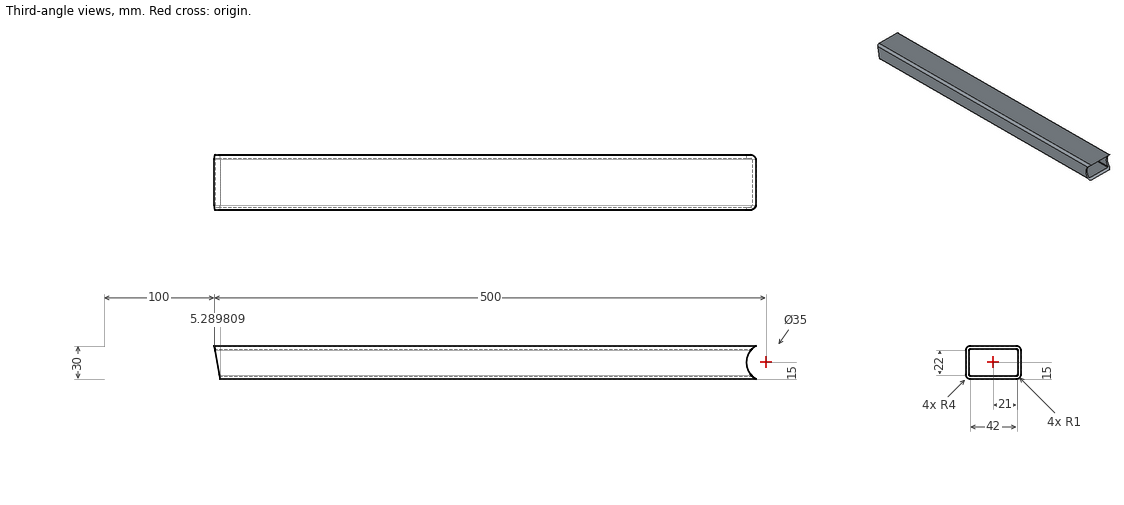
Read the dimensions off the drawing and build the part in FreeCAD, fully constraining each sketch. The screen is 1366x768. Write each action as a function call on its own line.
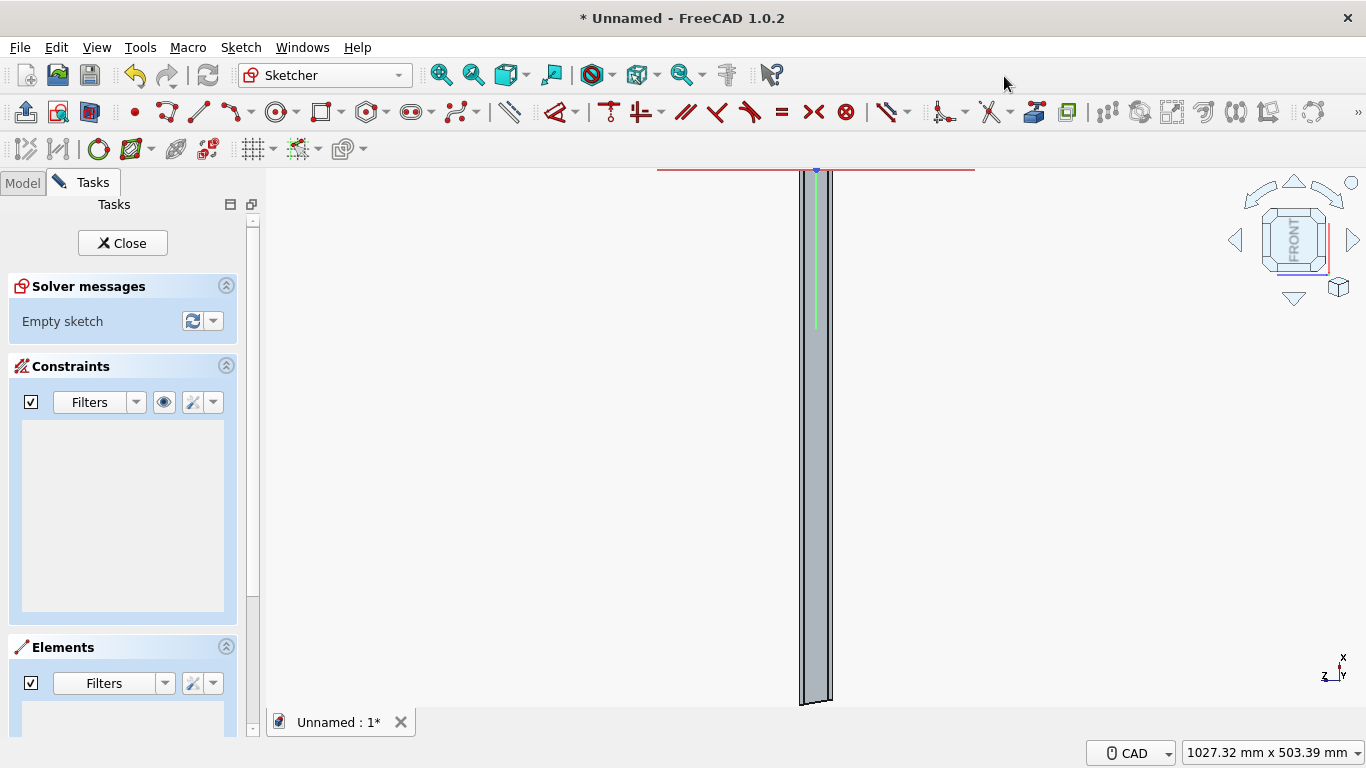
scroll(748, 438, down, 5)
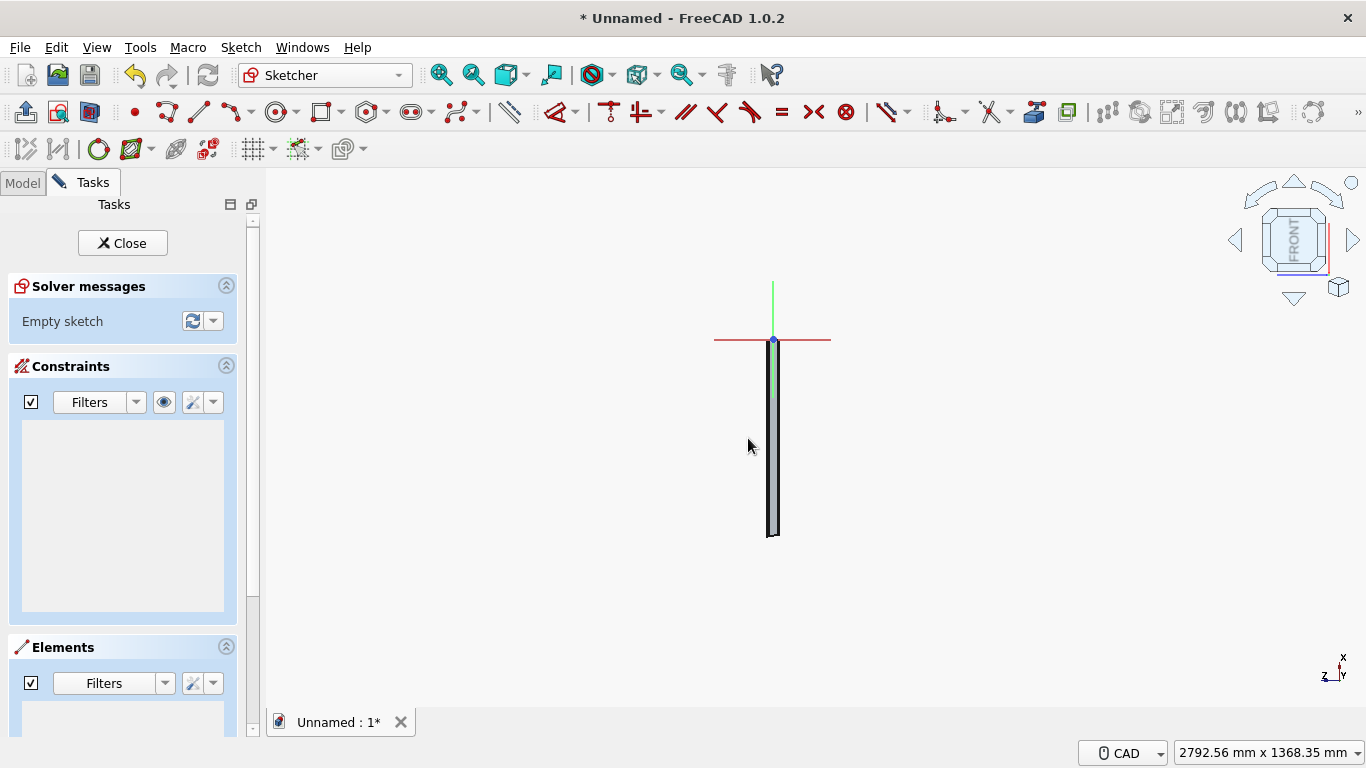
scroll(775, 335, up, 15)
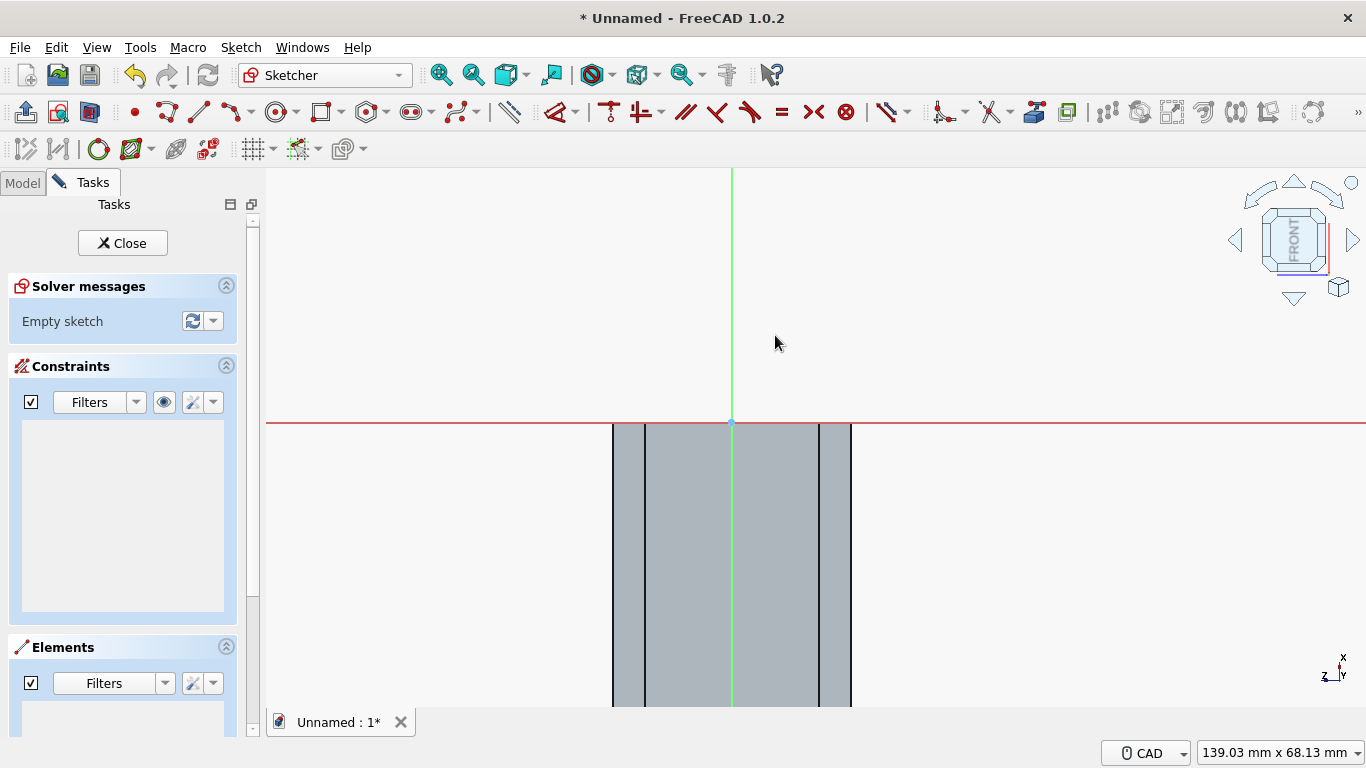
key(g)
key(c)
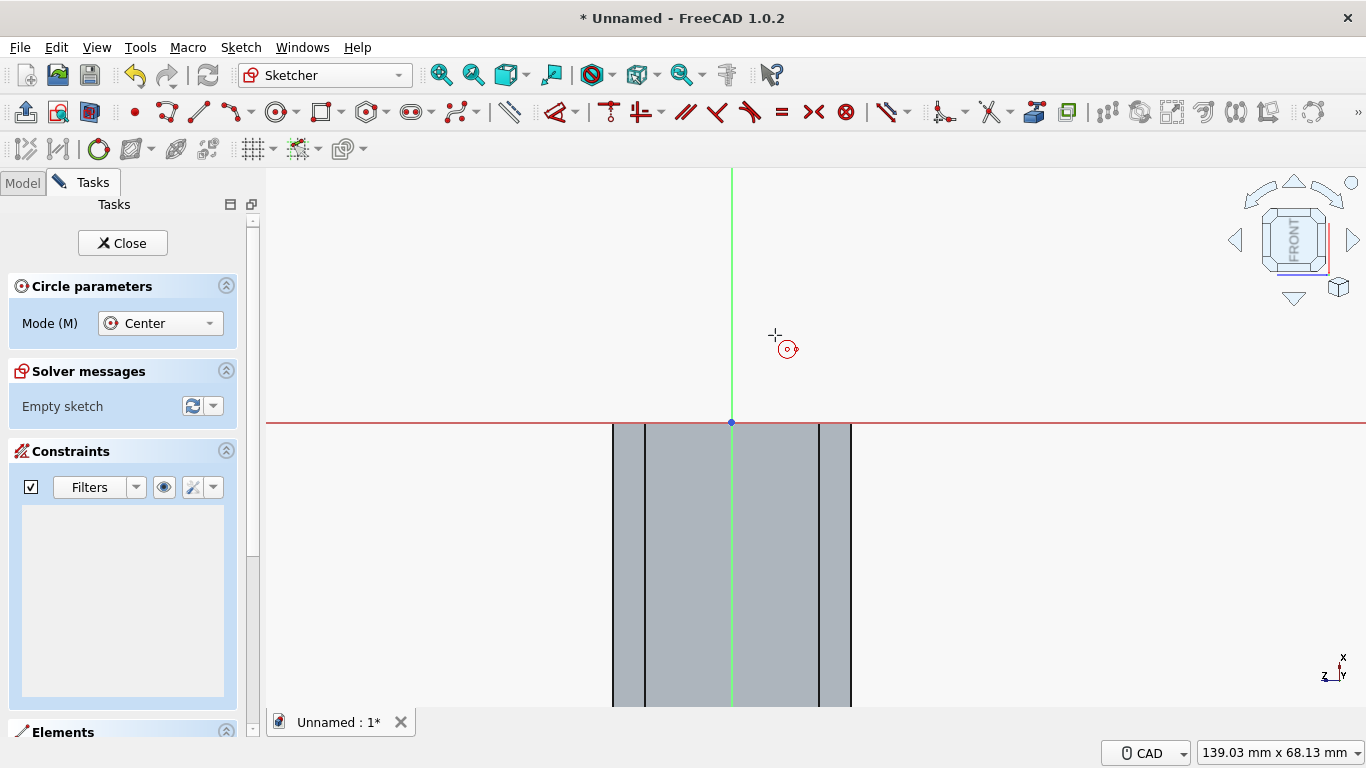
click(732, 423)
click(830, 325)
key(Escape)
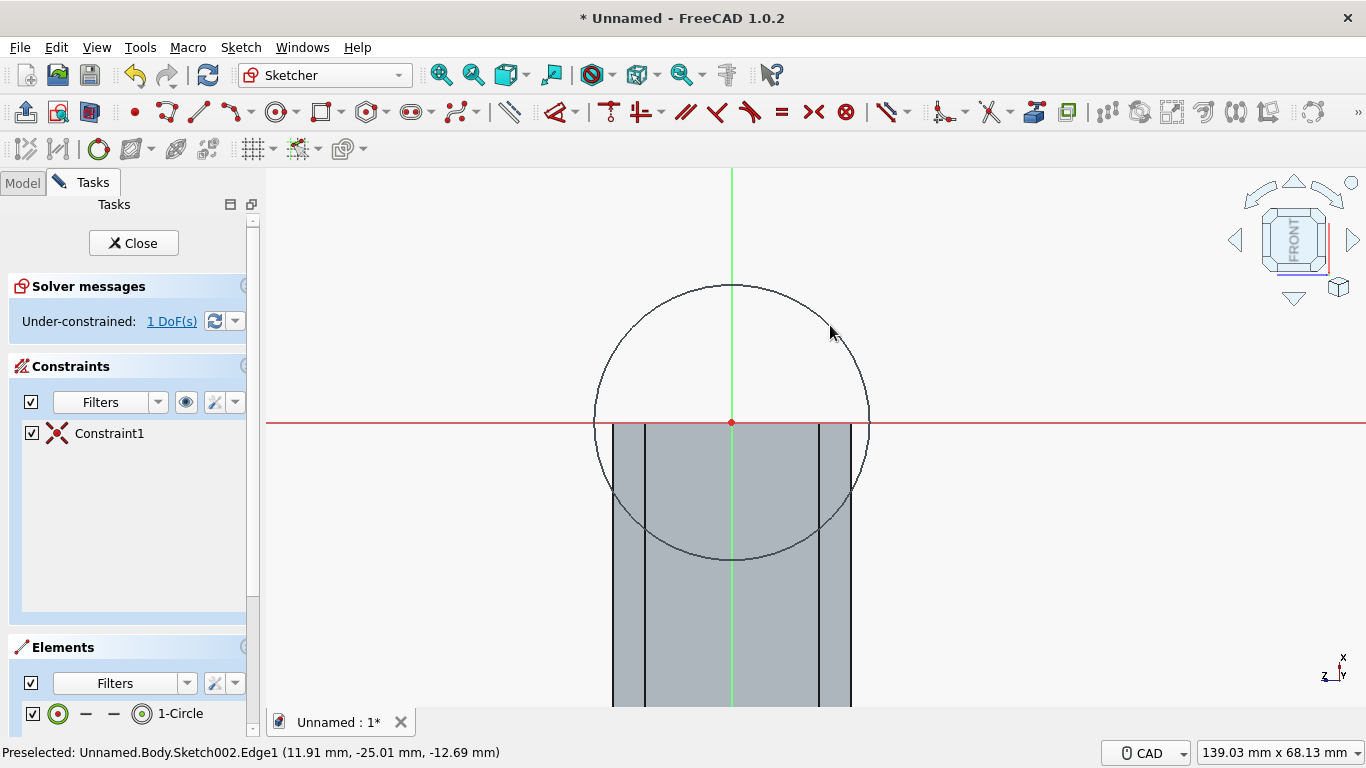
key(d)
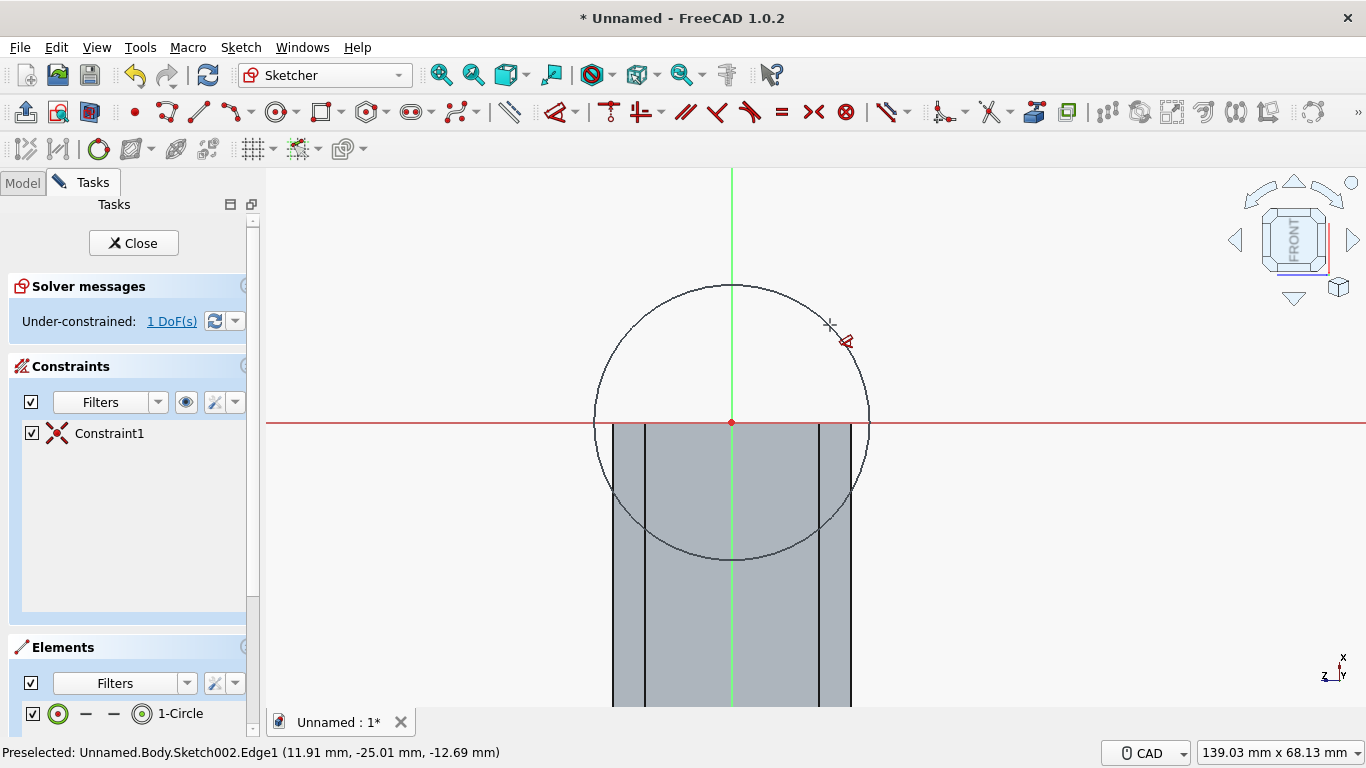
click(829, 325)
click(852, 302)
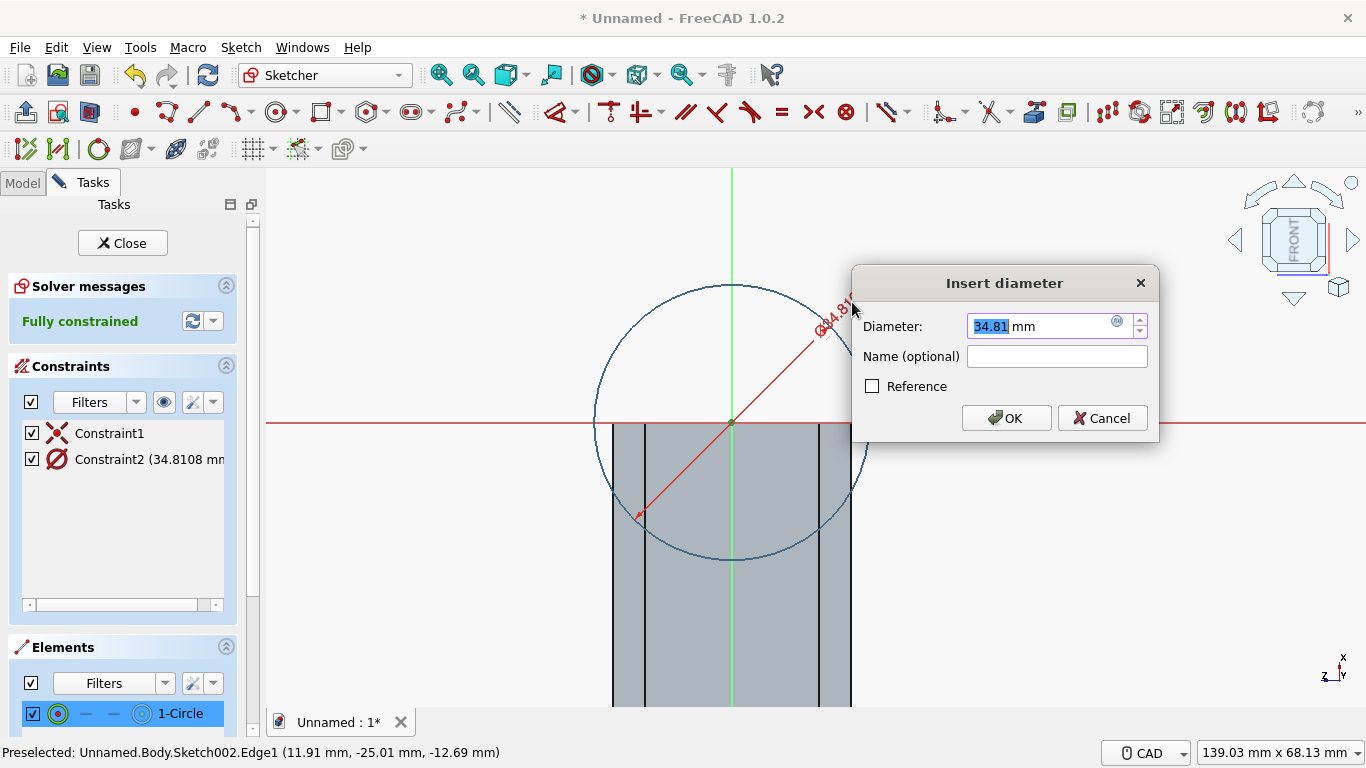
text(35)
key(Return)
key(Escape)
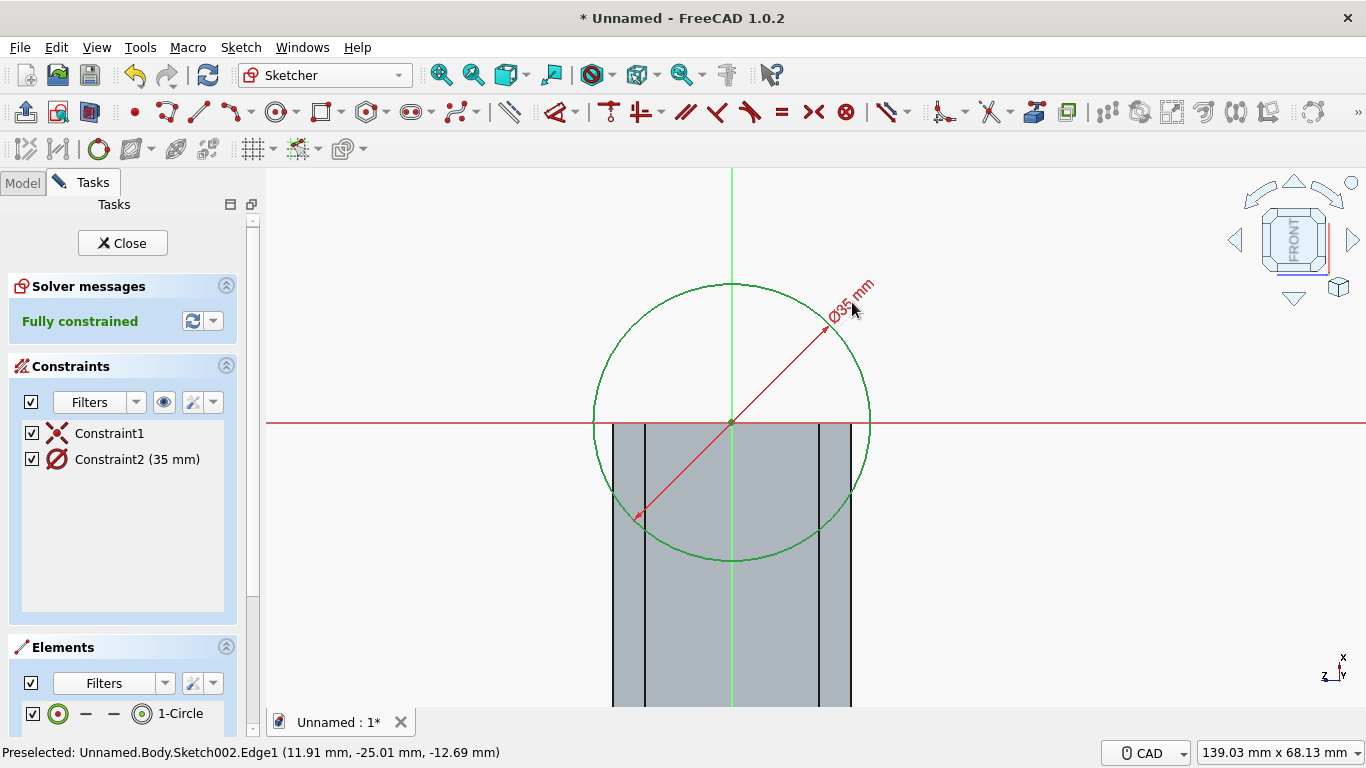
click(123, 243)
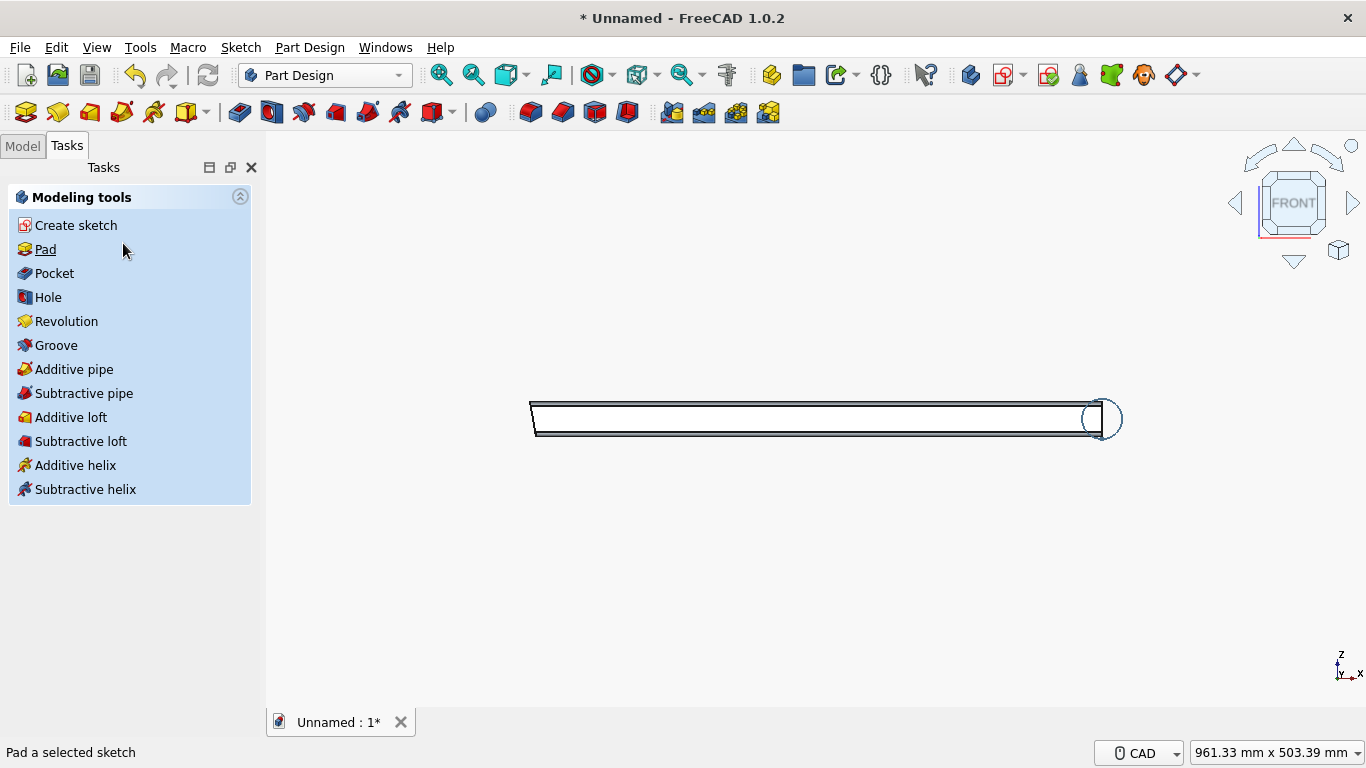
click(240, 112)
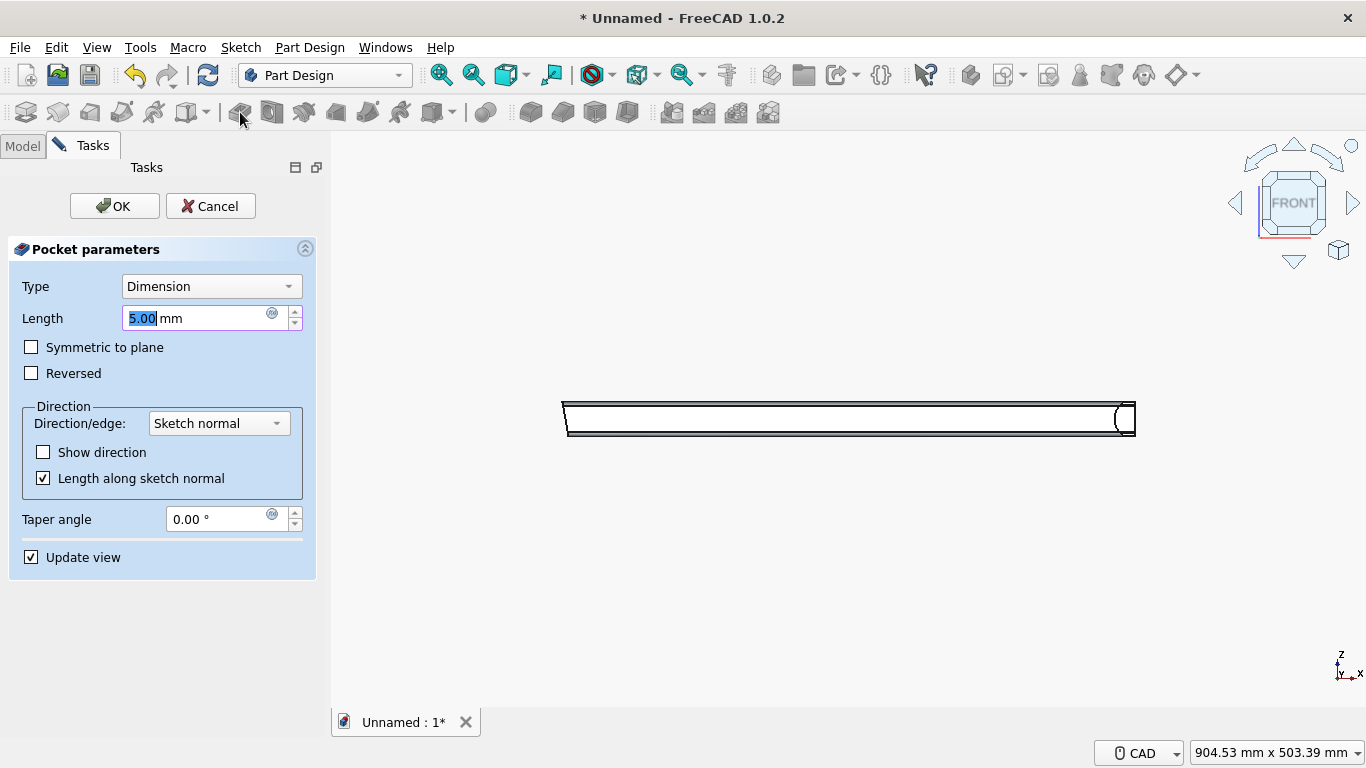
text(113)
key(Tab)